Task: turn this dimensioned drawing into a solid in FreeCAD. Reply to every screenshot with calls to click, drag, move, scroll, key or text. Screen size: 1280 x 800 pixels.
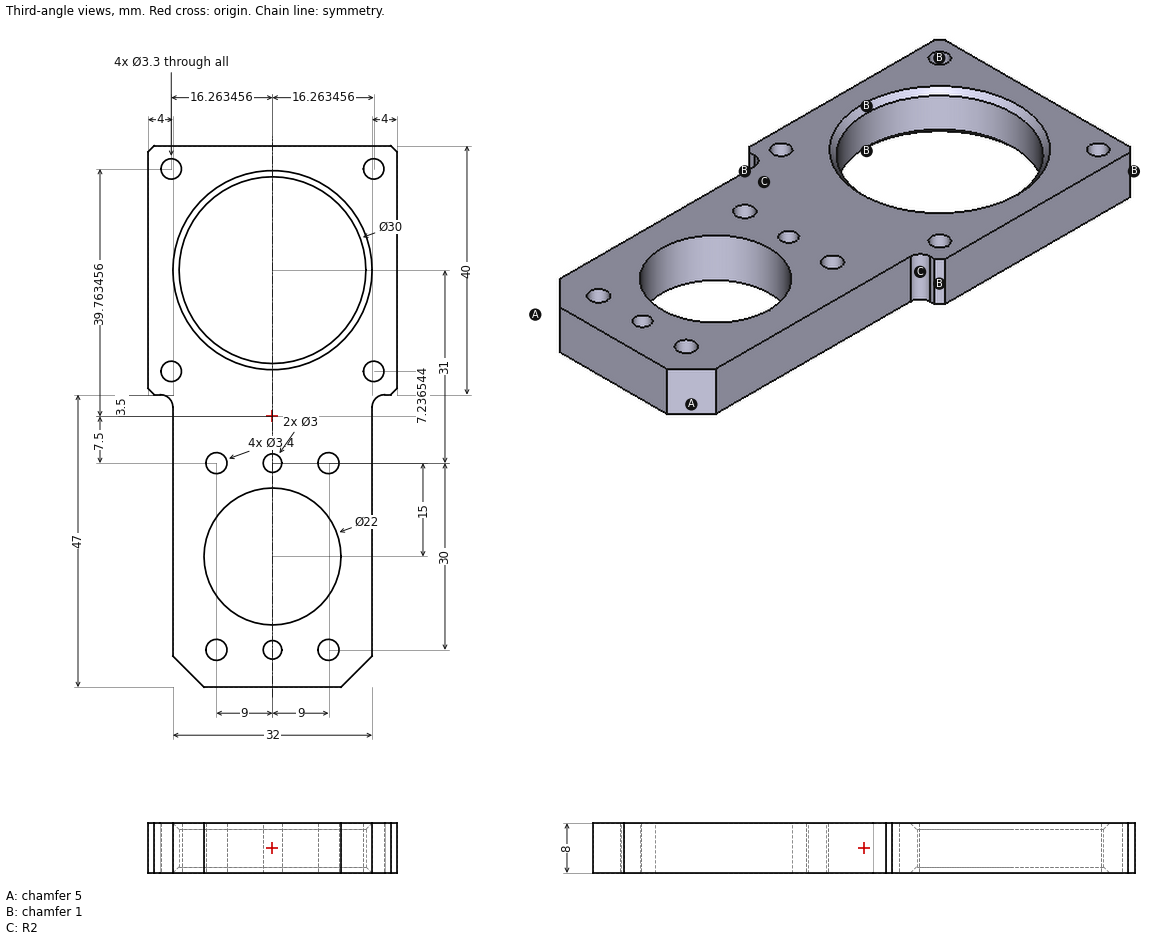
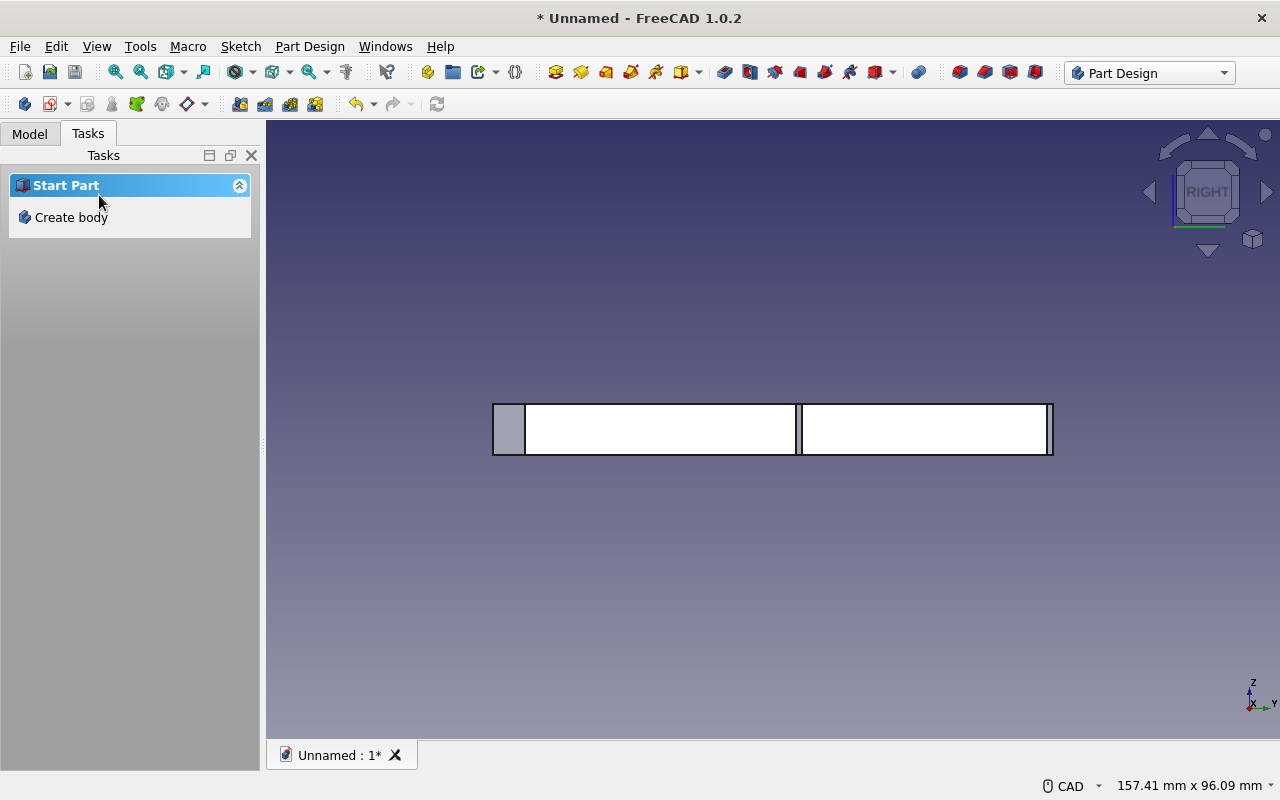
key(5)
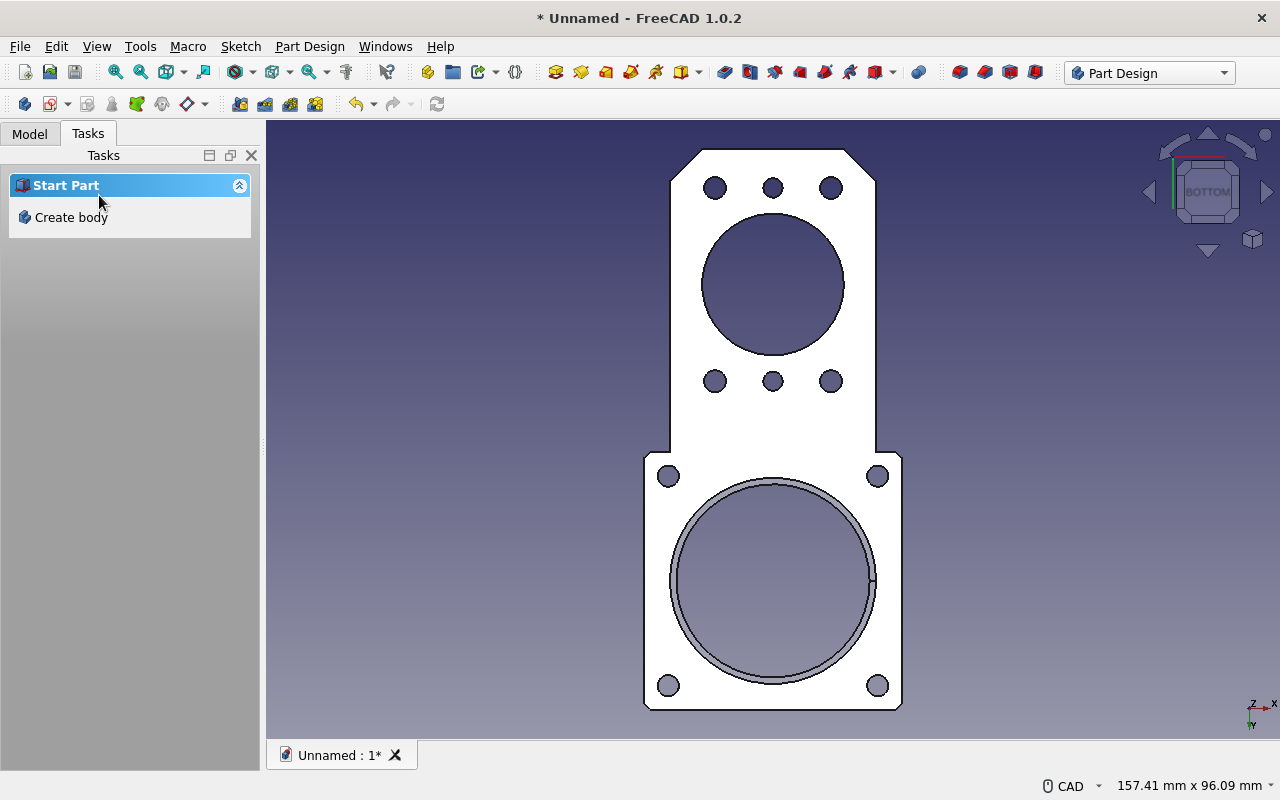
key(4)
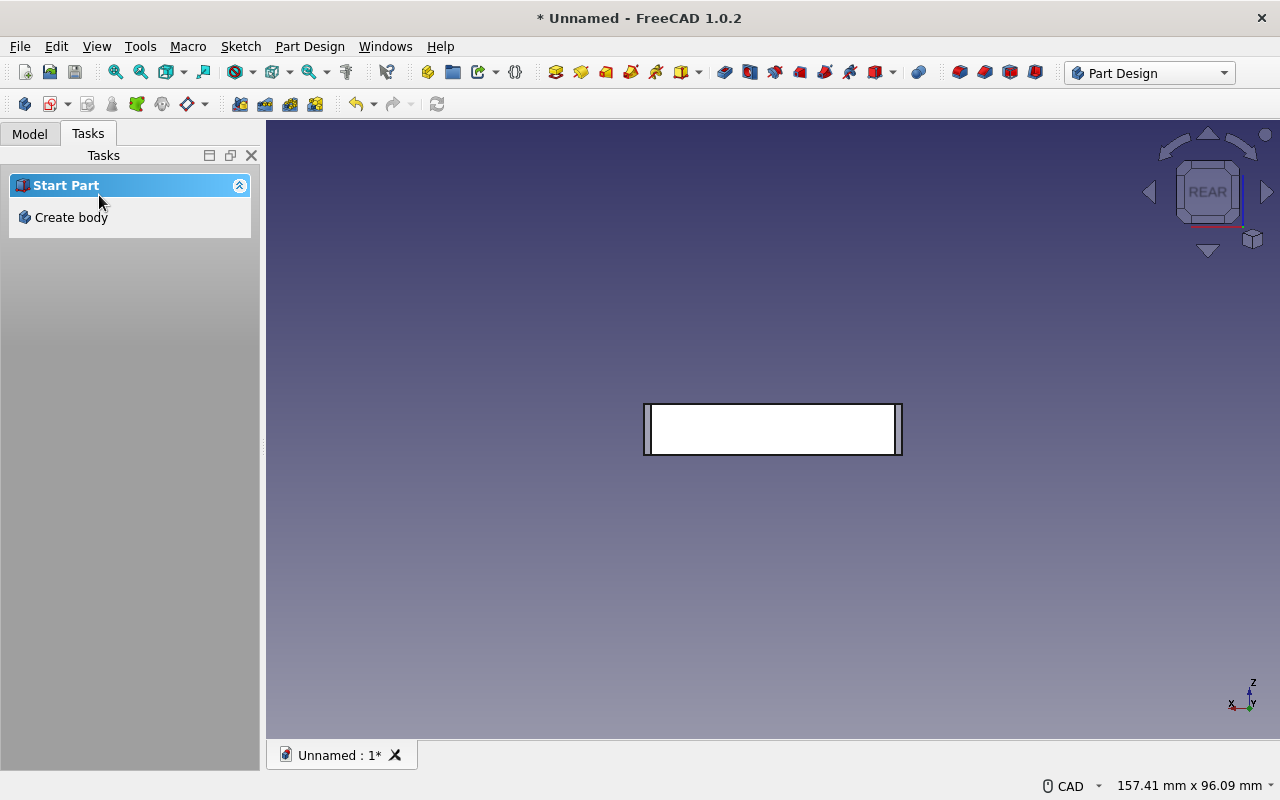
click(116, 72)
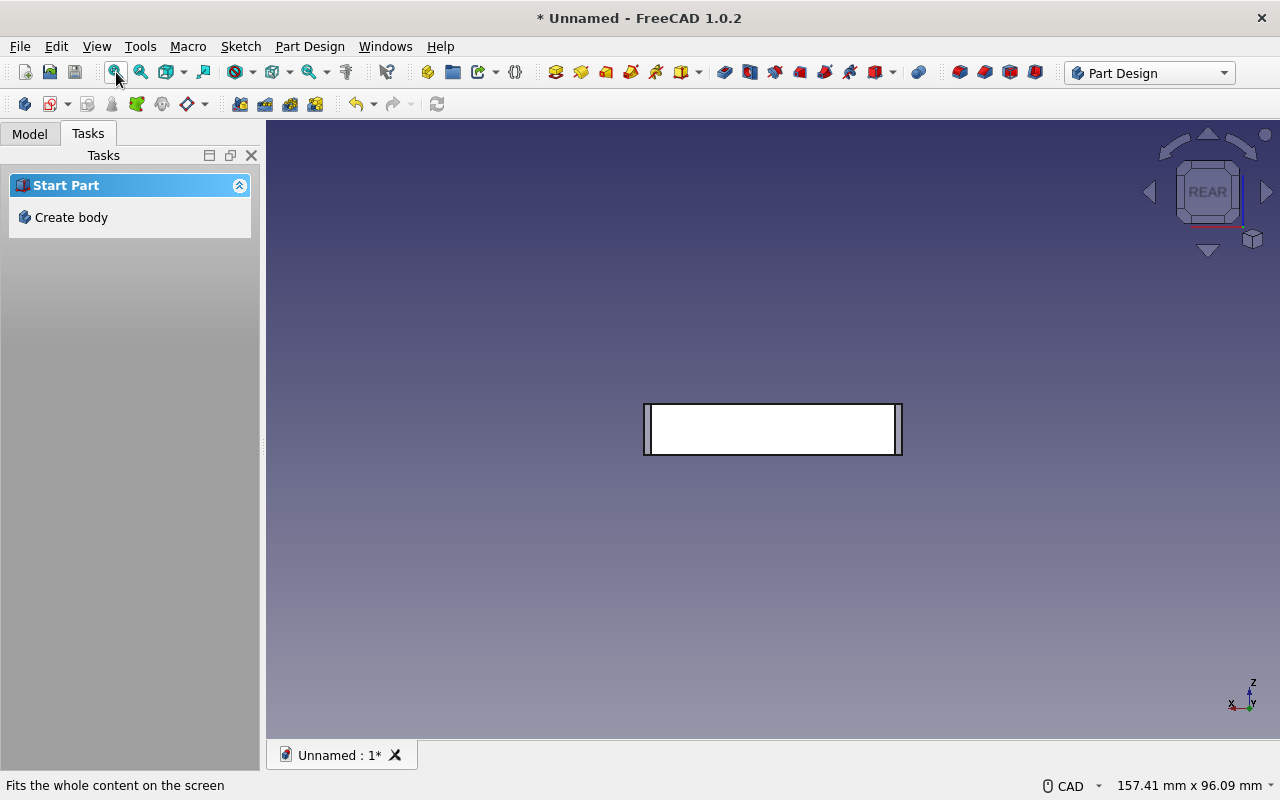
key(6)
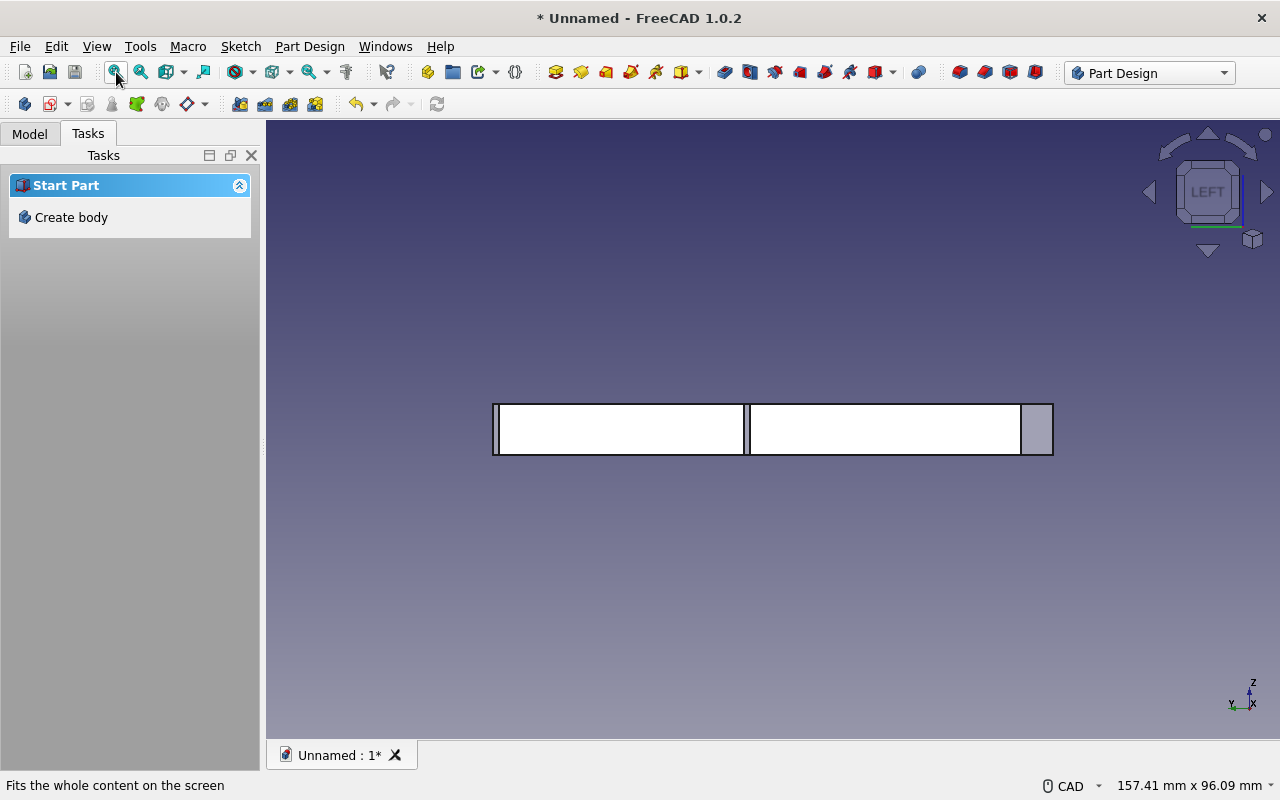
key(v)
key(3)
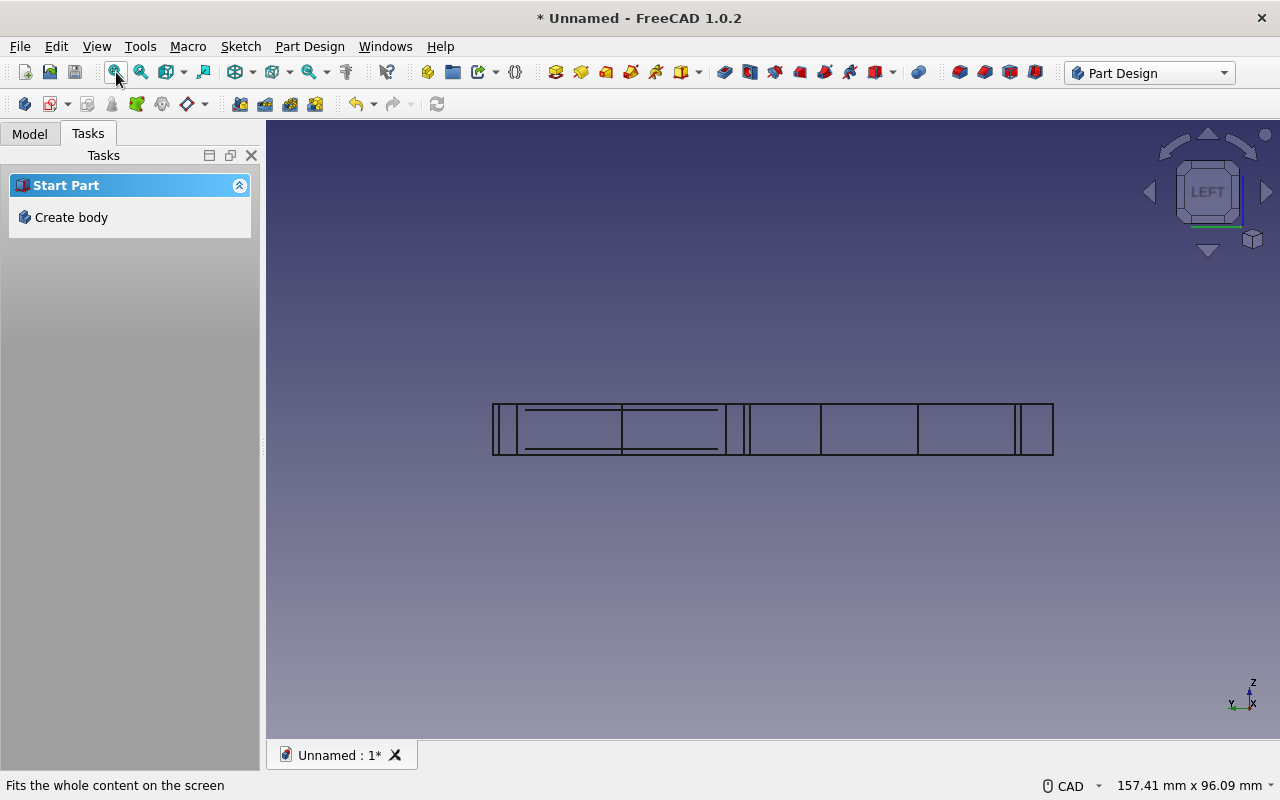
key(0)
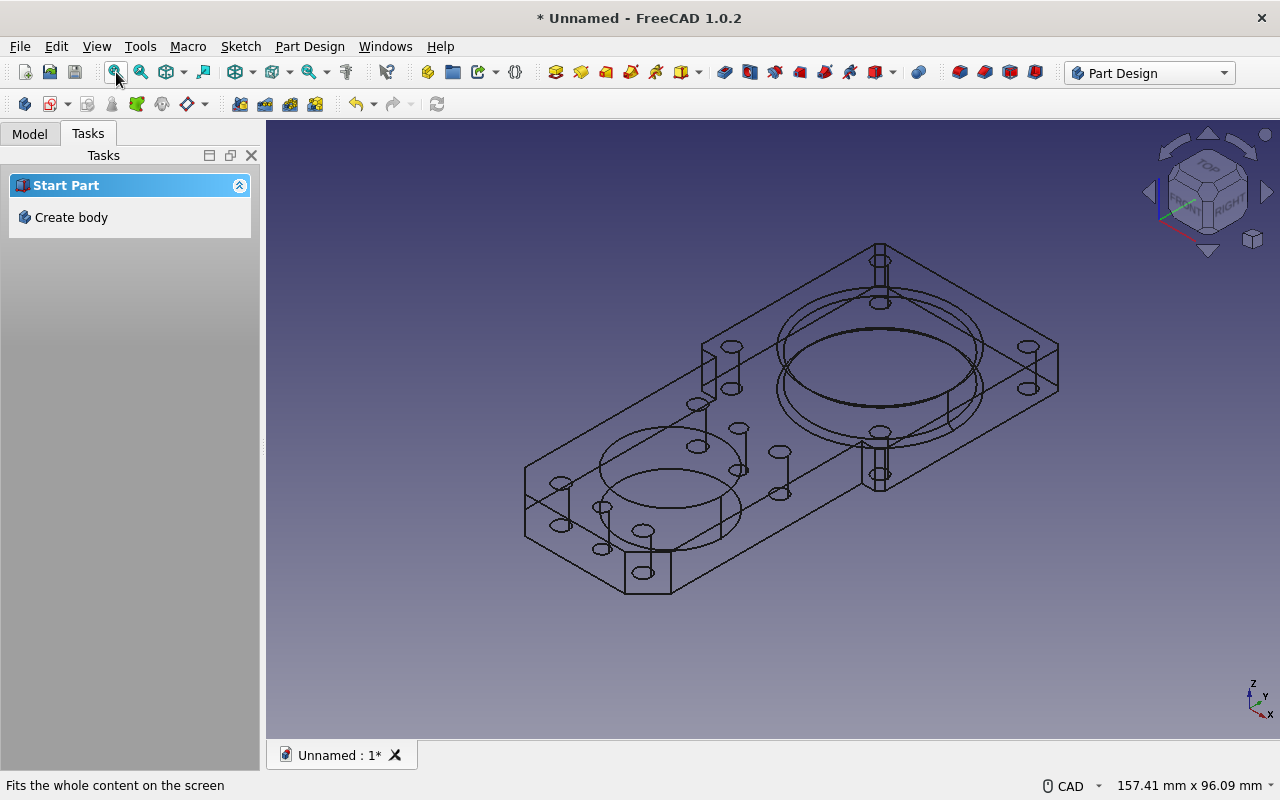
click(716, 377)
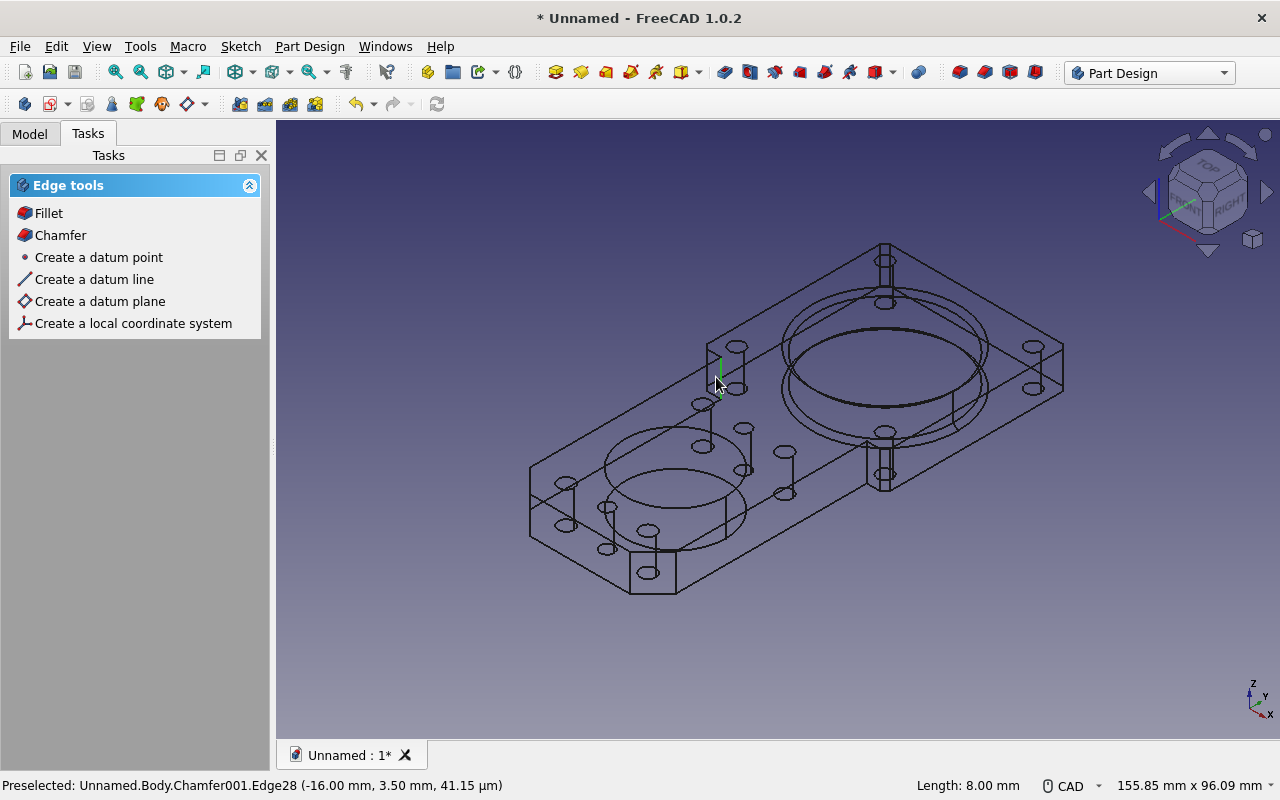
click(867, 461, ctrl)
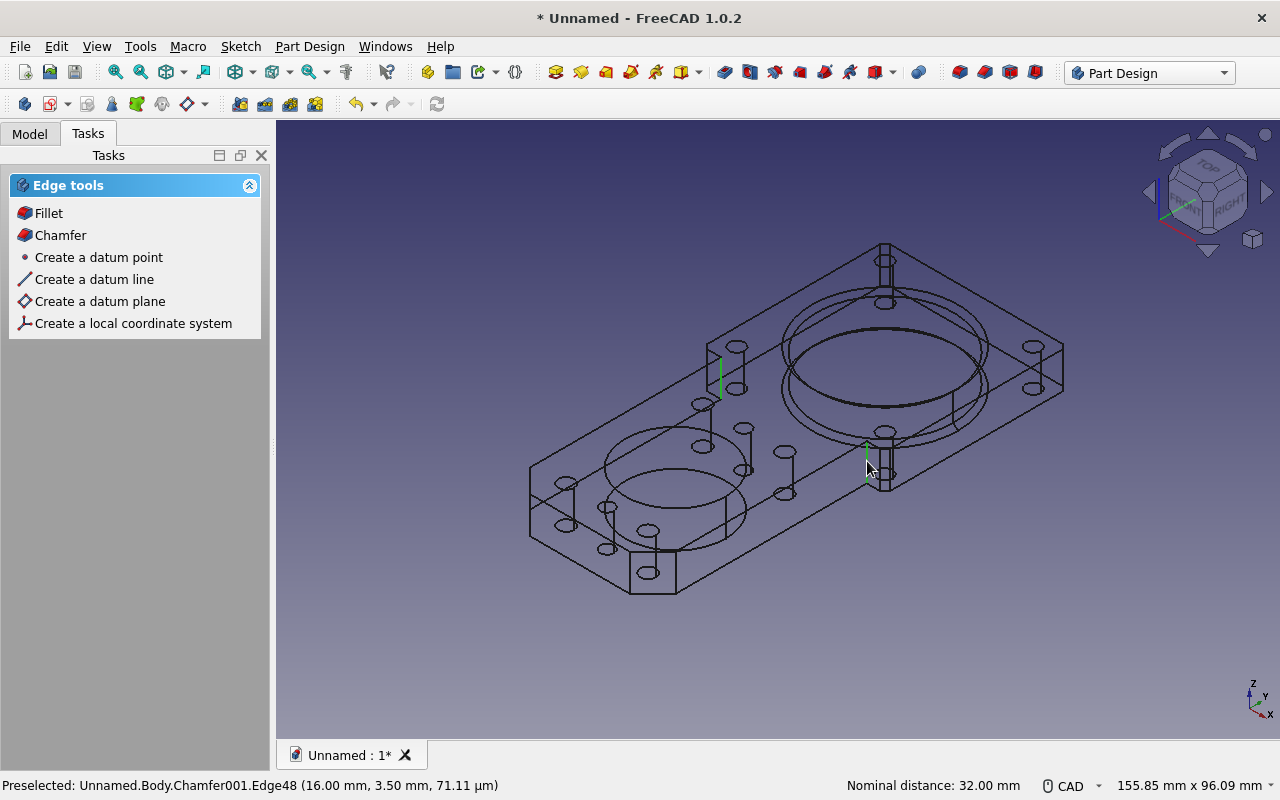
key(v)
key(1)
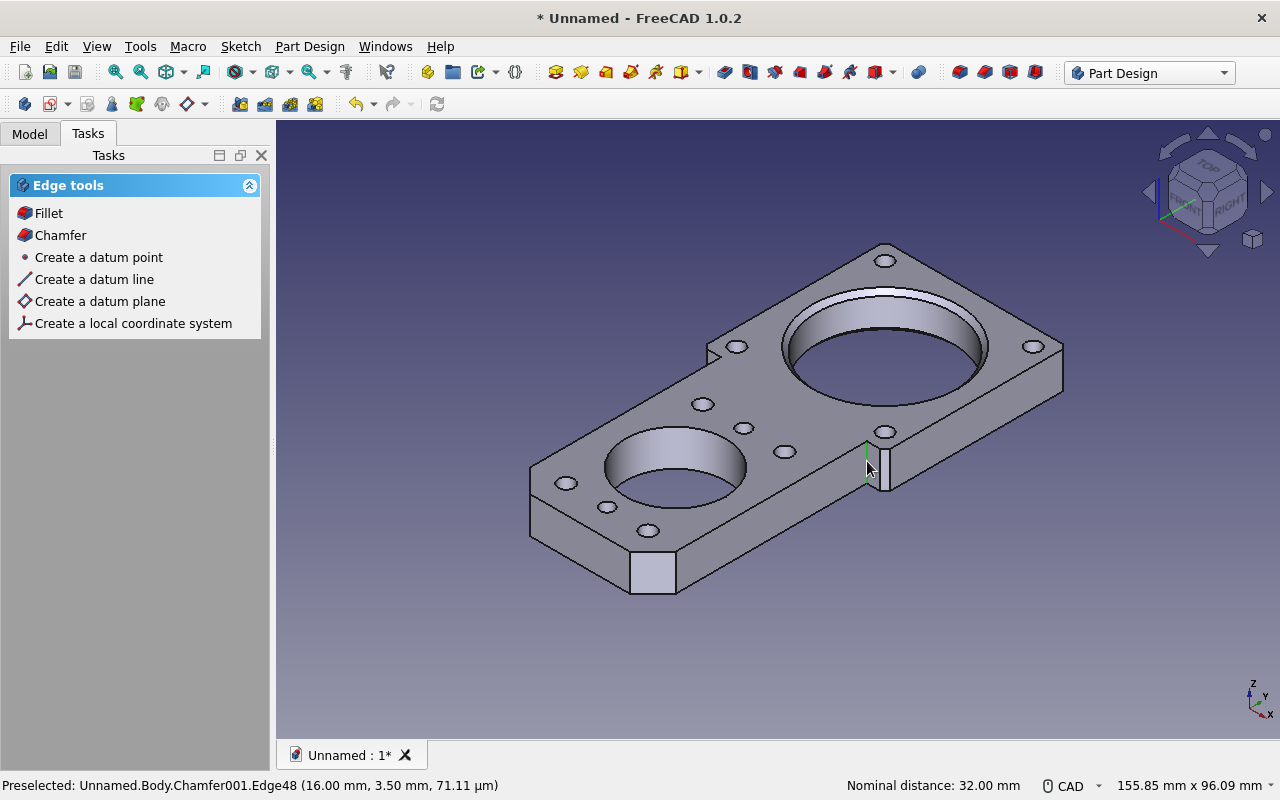
click(960, 72)